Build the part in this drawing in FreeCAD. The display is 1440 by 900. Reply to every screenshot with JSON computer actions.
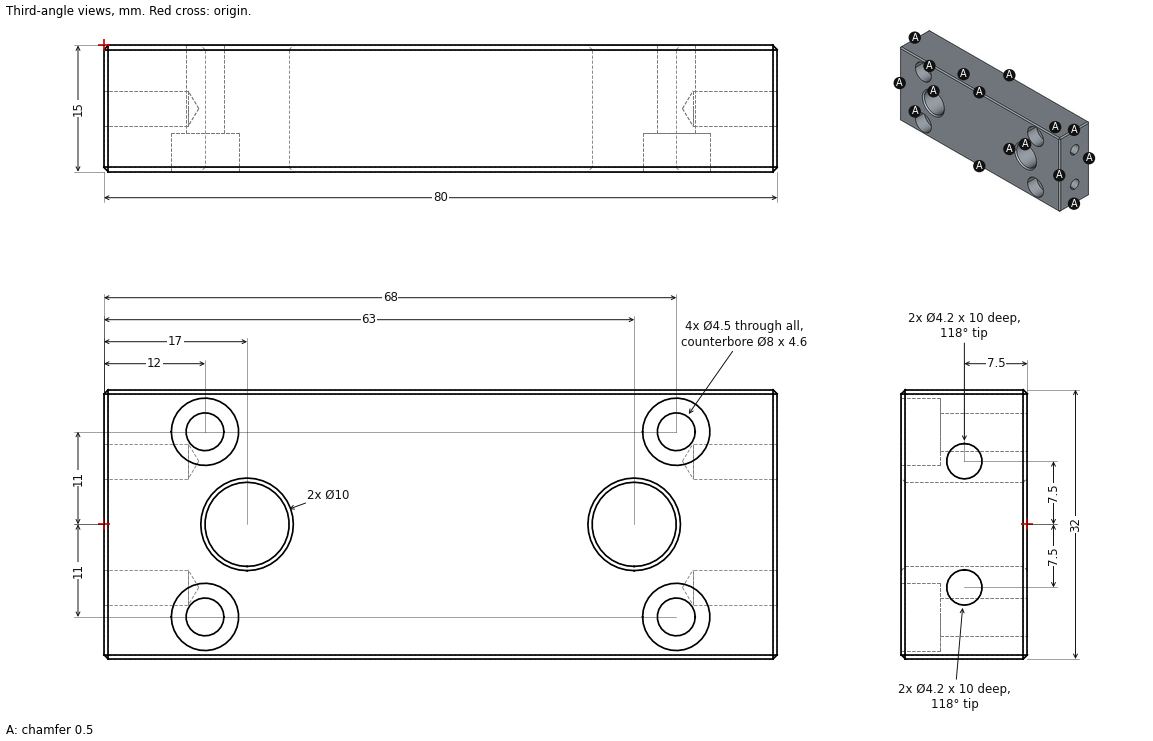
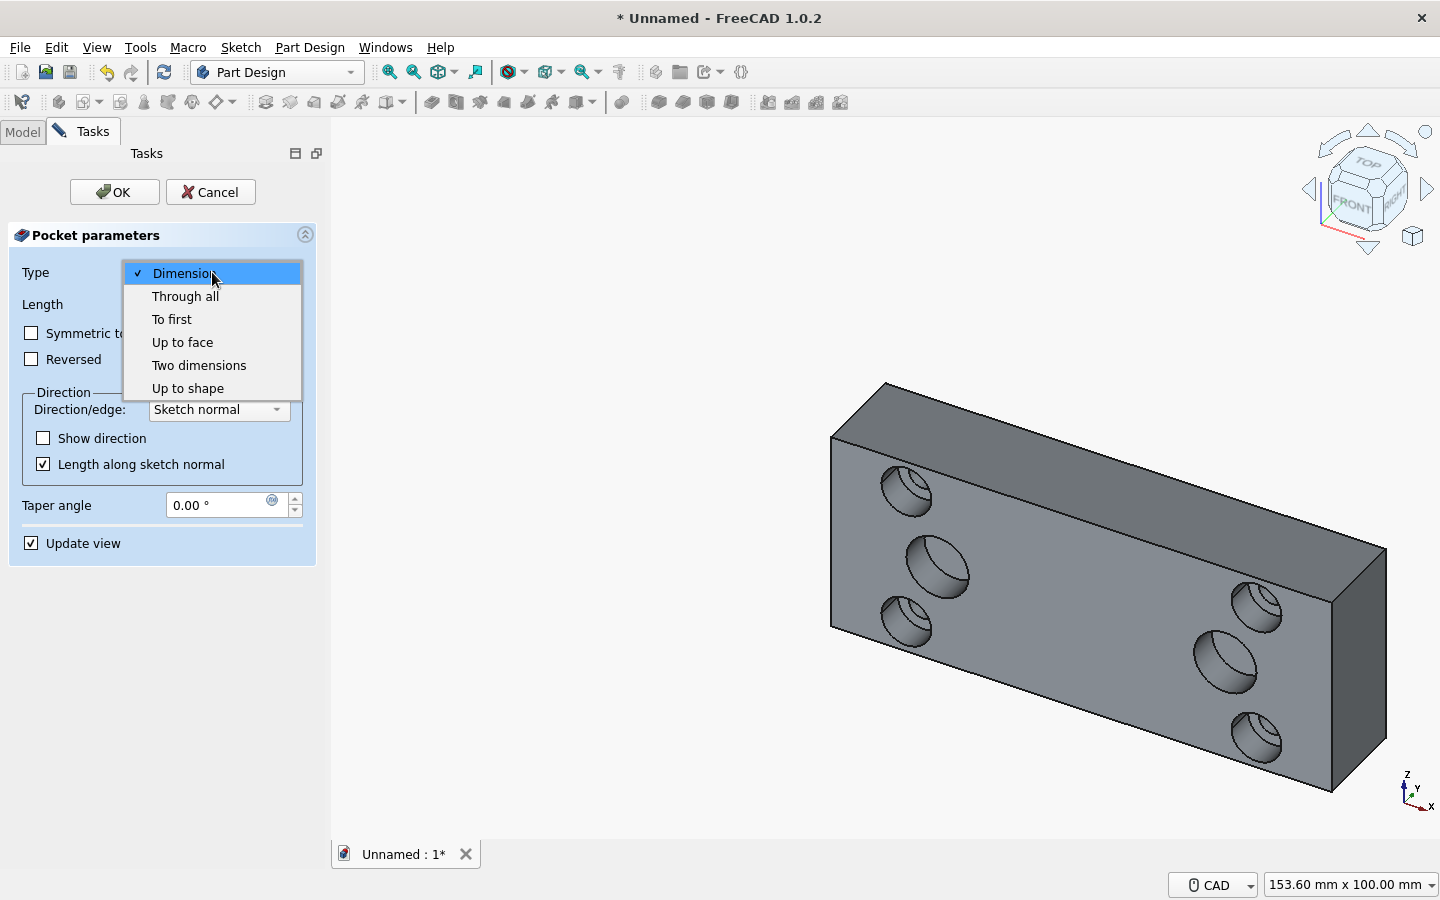
{"action": "left_click", "coordinate": [212, 296]}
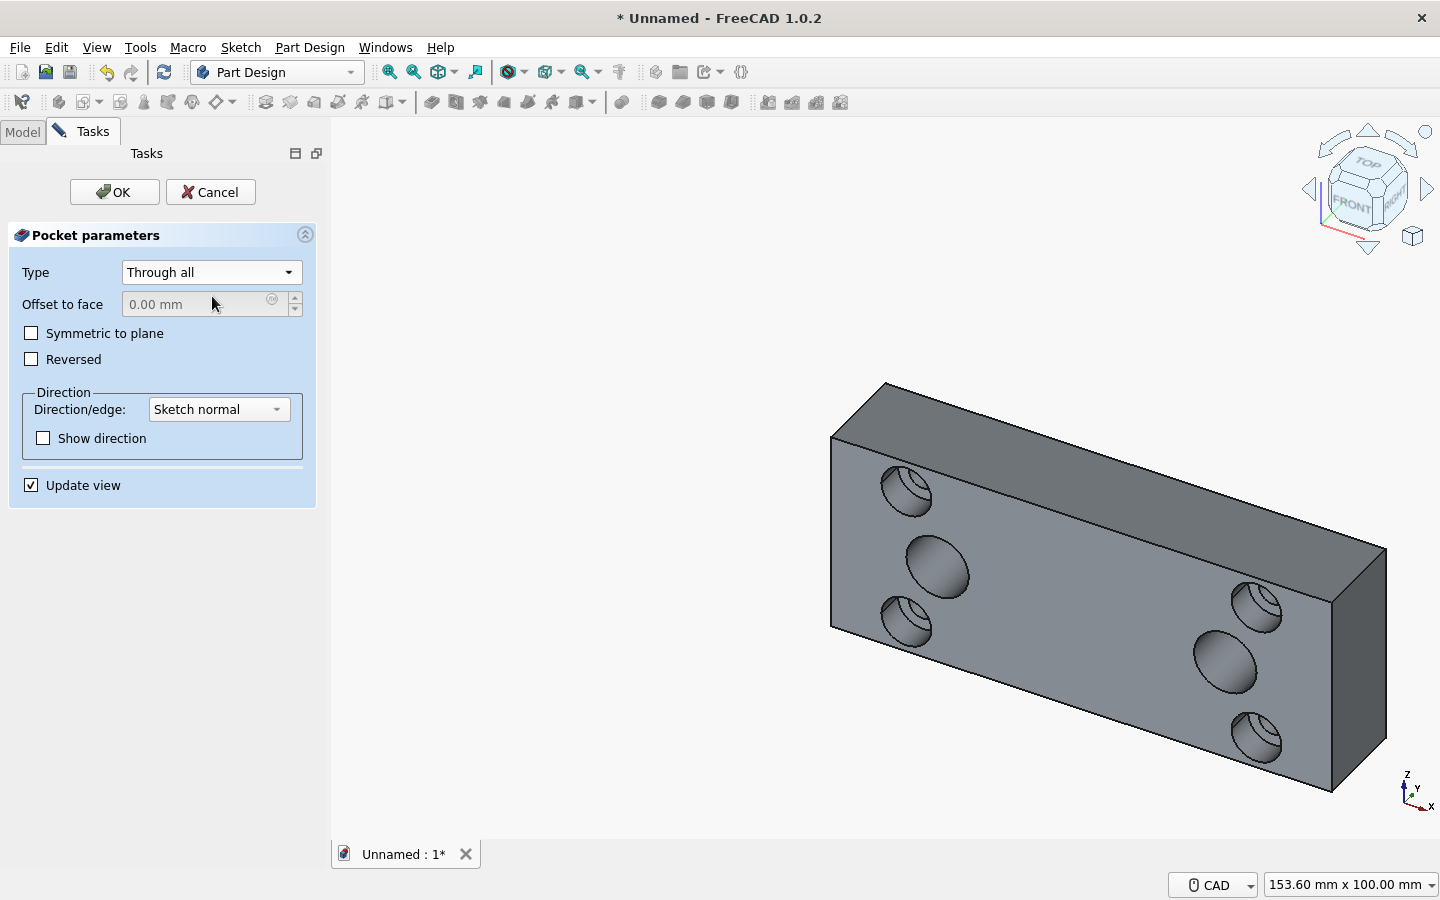
{"action": "left_click", "coordinate": [115, 192]}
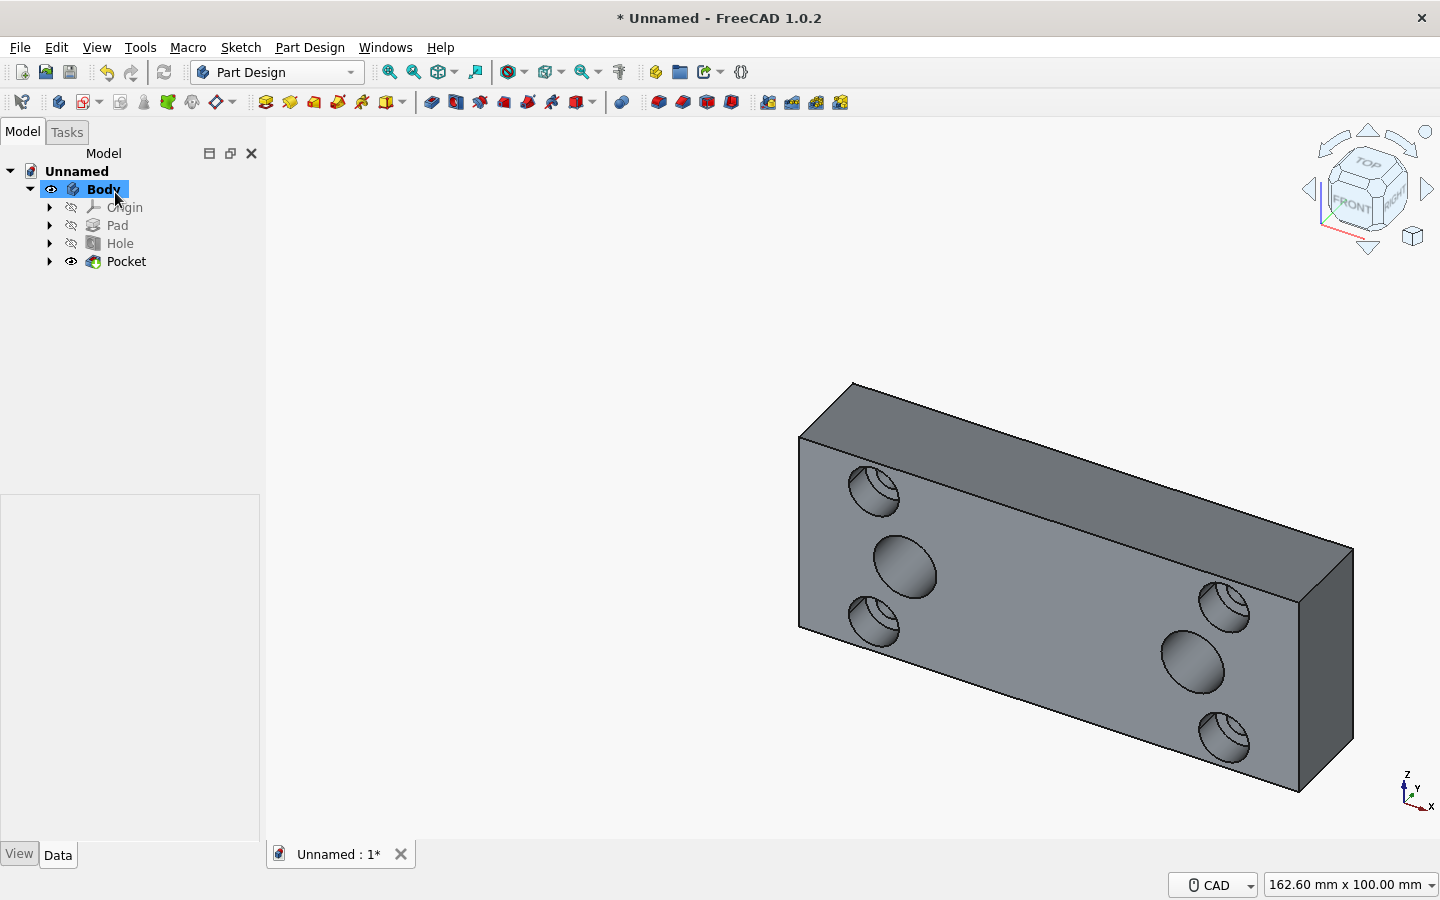
{"action": "left_click", "coordinate": [1326, 643]}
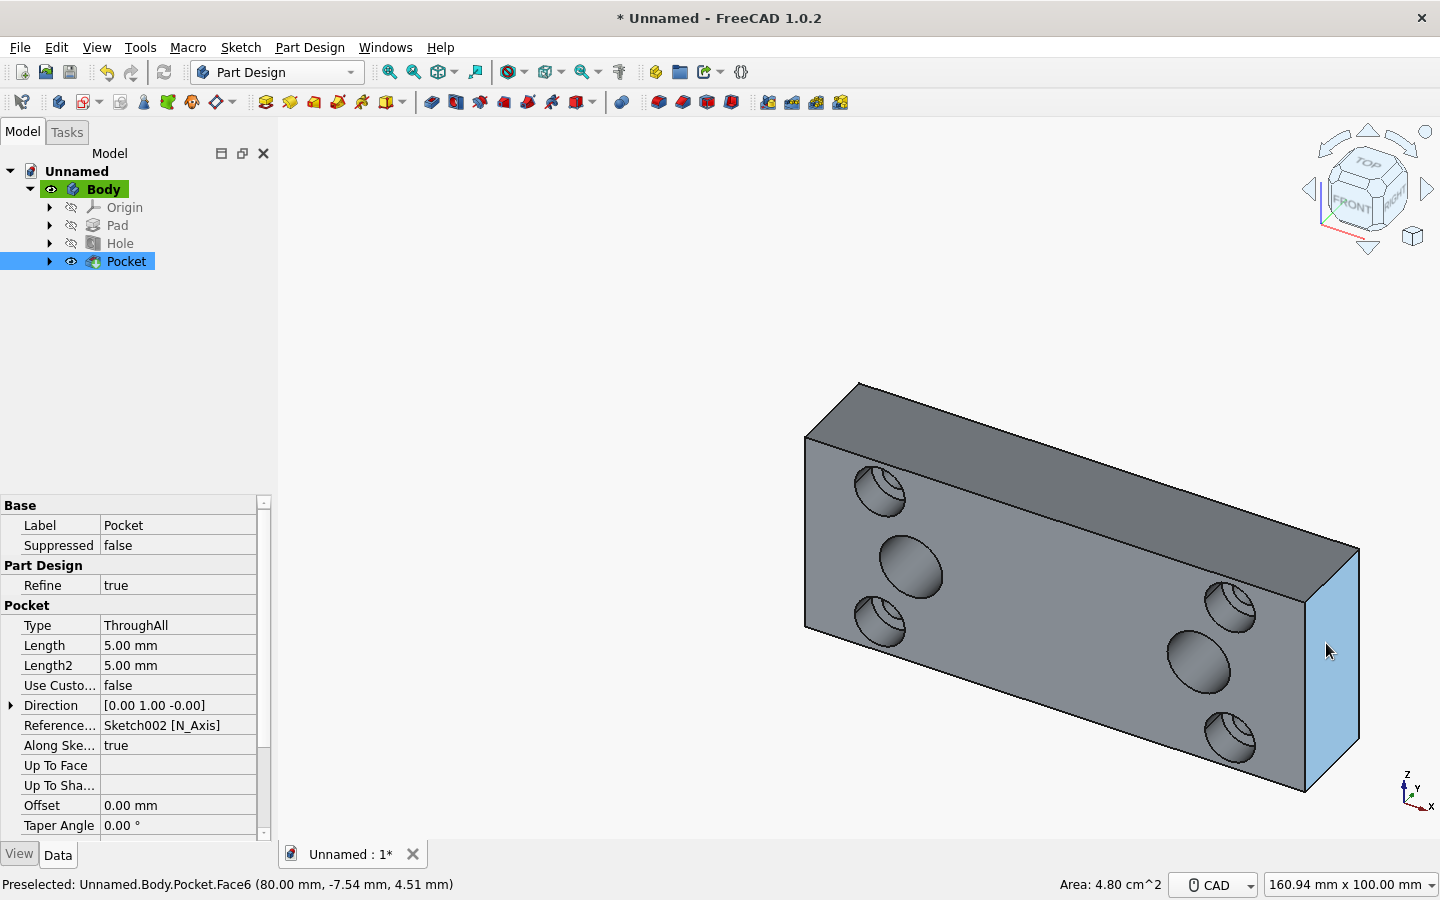
{"action": "left_click", "coordinate": [84, 102]}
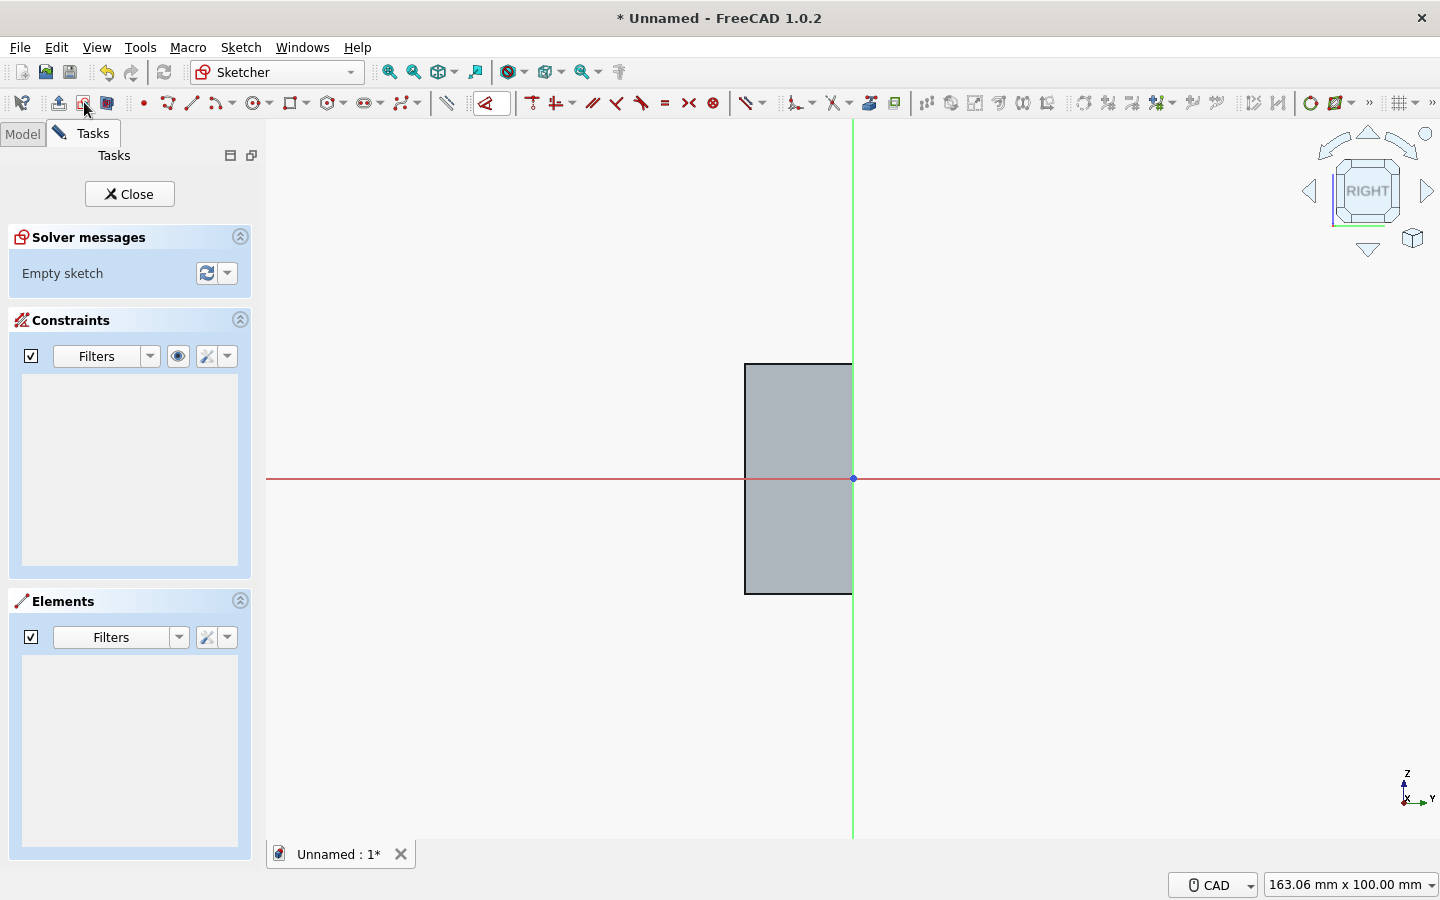
{"action": "scroll", "coordinate": [833, 479], "scroll_direction": "up", "scroll_amount": 6}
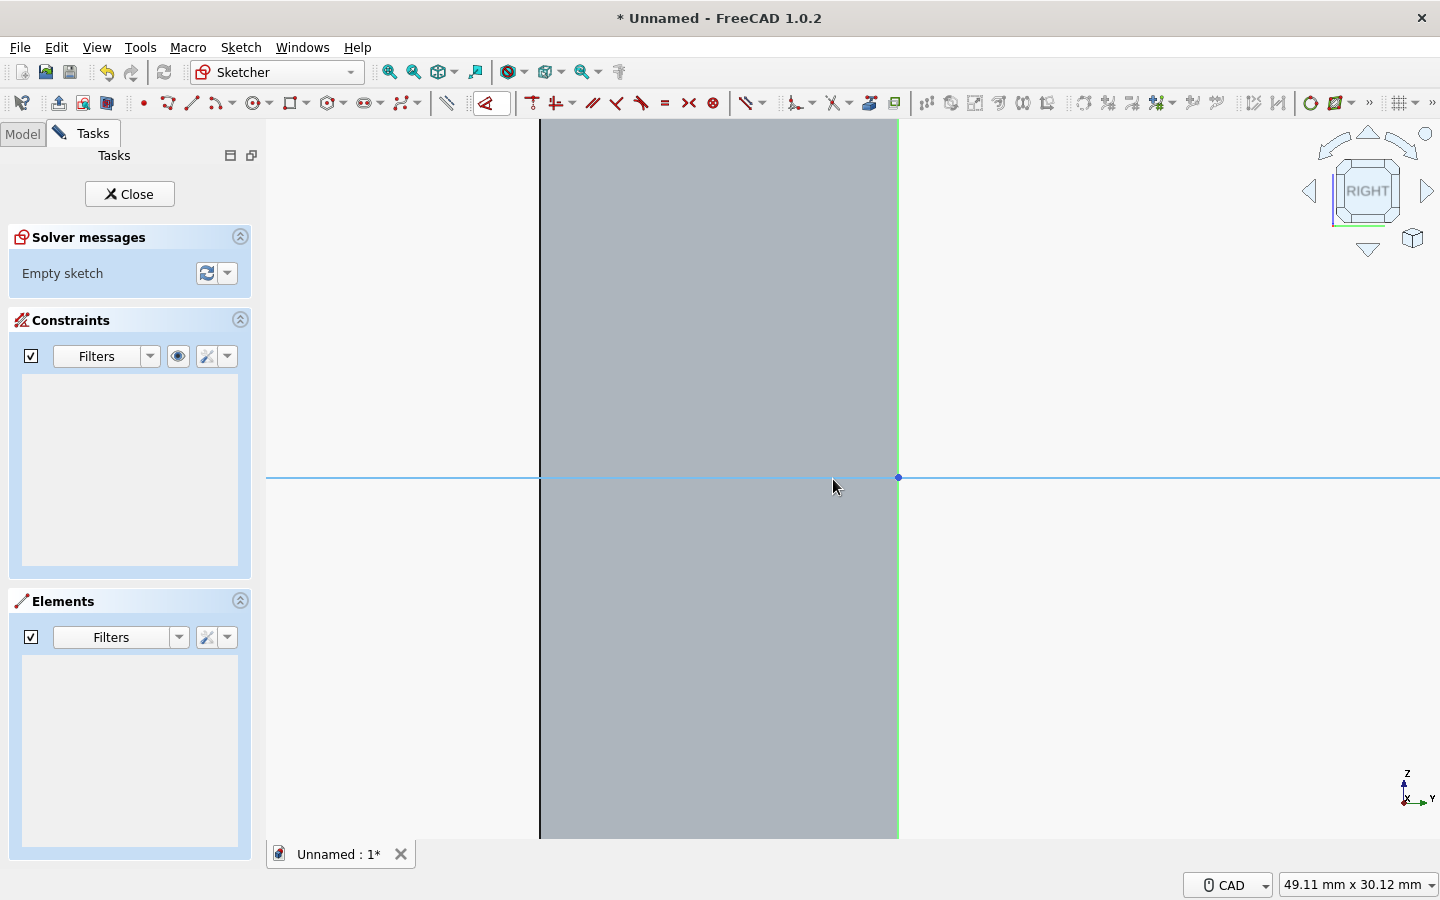
{"action": "left_click", "coordinate": [254, 104]}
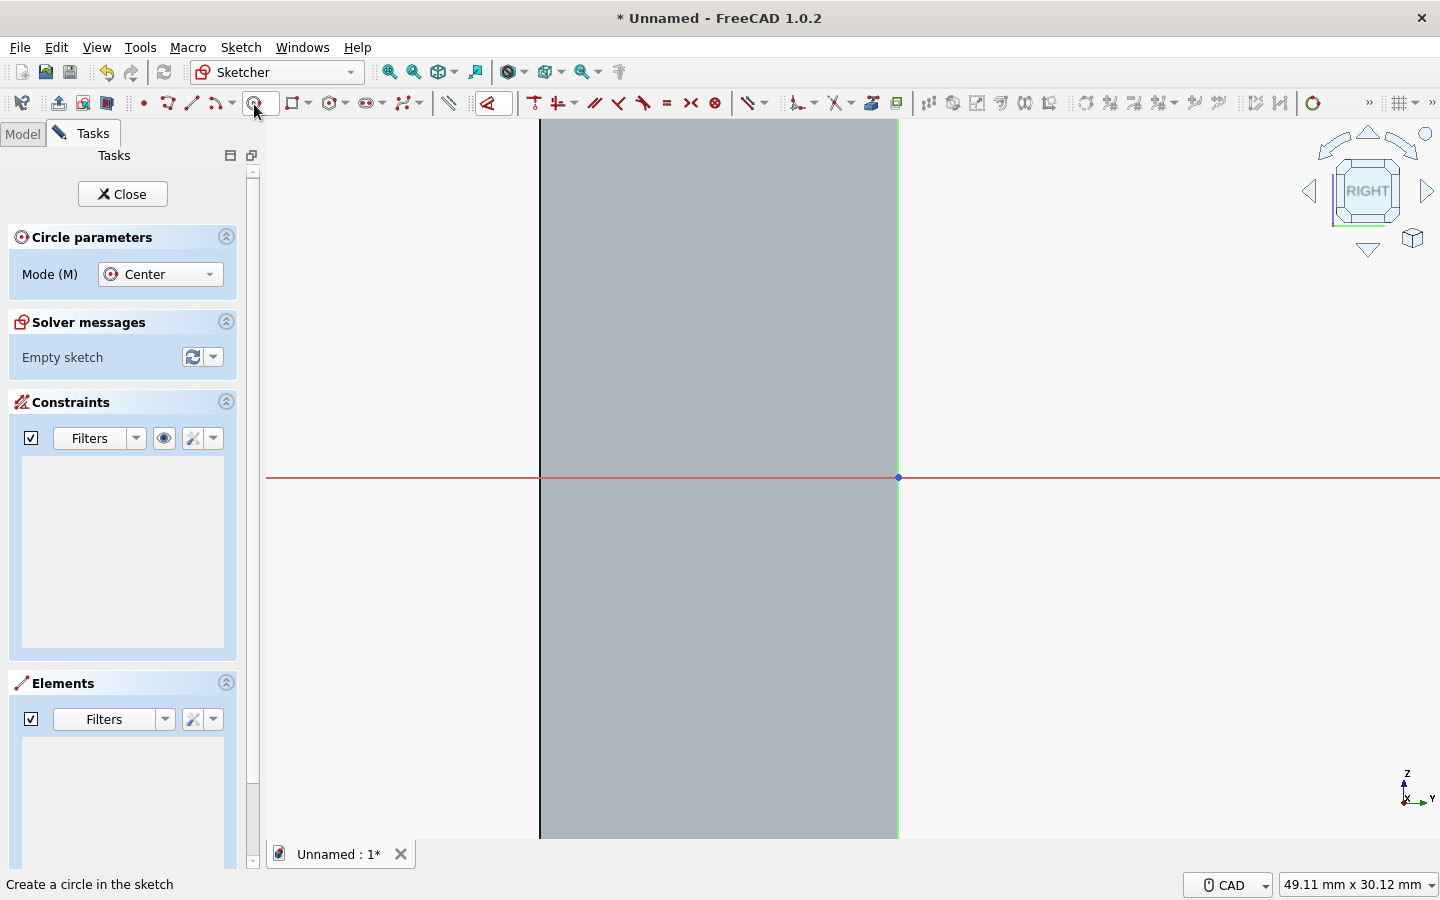
{"action": "left_click", "coordinate": [719, 299]}
{"action": "left_click", "coordinate": [754, 263]}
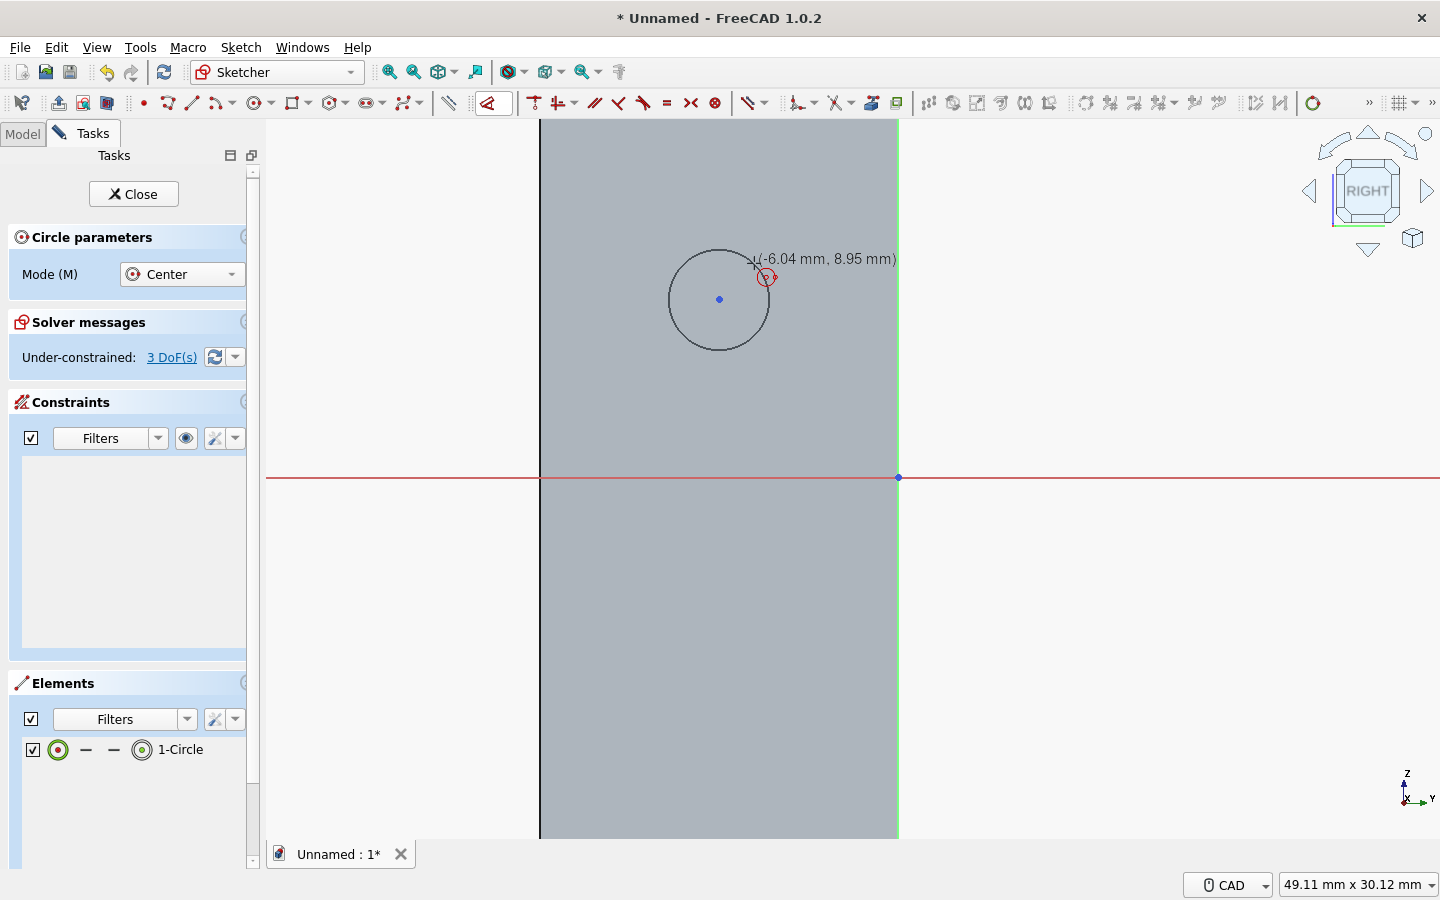
{"action": "left_click", "coordinate": [719, 657]}
{"action": "left_click", "coordinate": [754, 622]}
{"action": "key", "text": "Escape"}